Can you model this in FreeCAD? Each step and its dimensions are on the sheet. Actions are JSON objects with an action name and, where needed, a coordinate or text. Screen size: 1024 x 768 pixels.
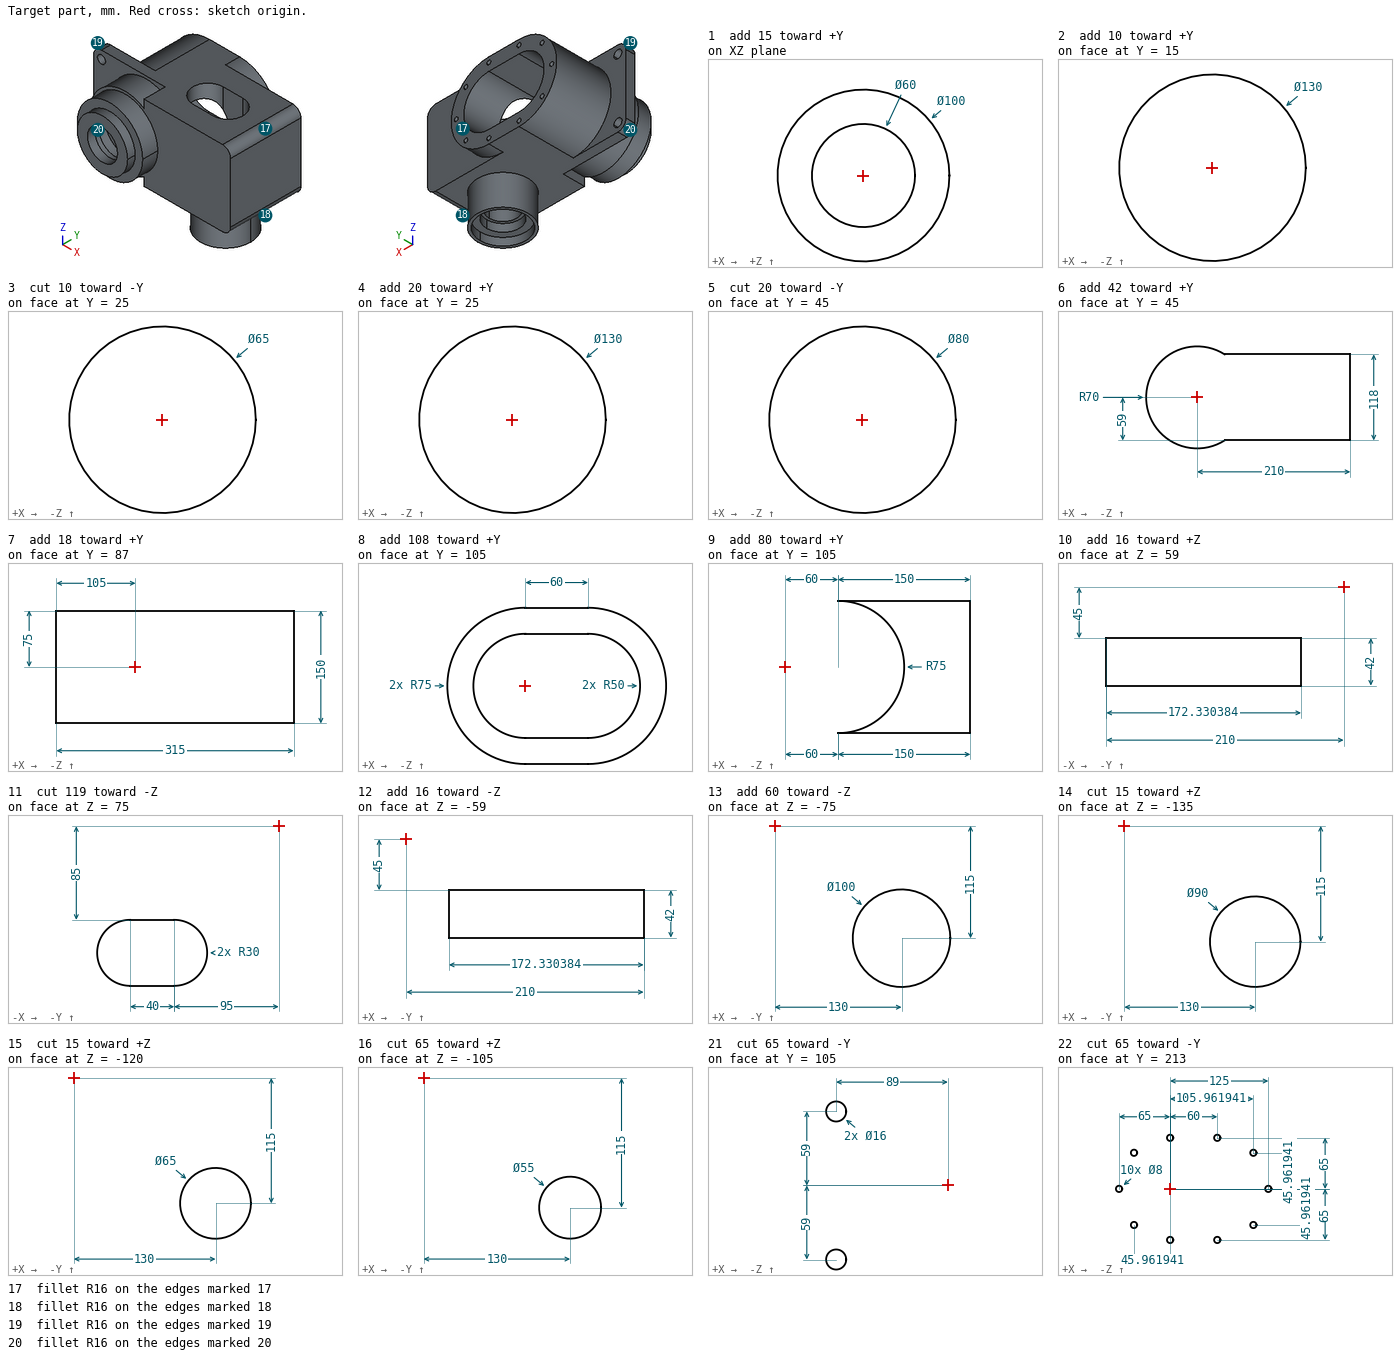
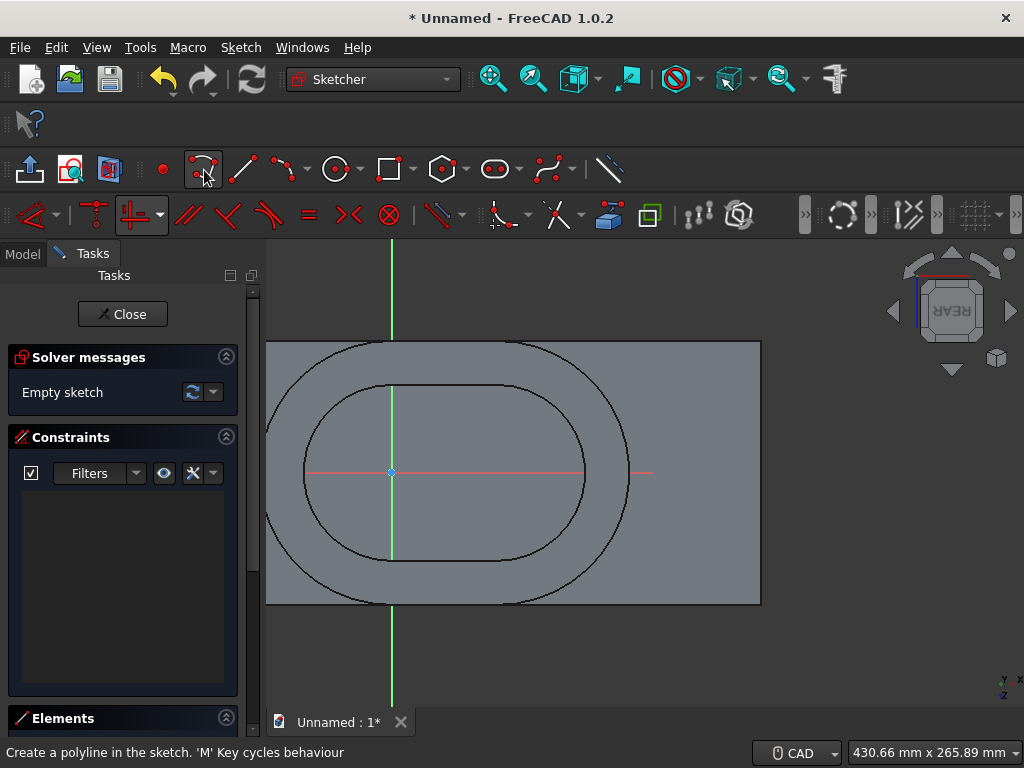
{"action": "left_click", "coordinate": [497, 605]}
{"action": "left_click", "coordinate": [761, 605]}
{"action": "left_click", "coordinate": [761, 341]}
{"action": "left_click", "coordinate": [497, 341]}
{"action": "right_click", "coordinate": [497, 341]}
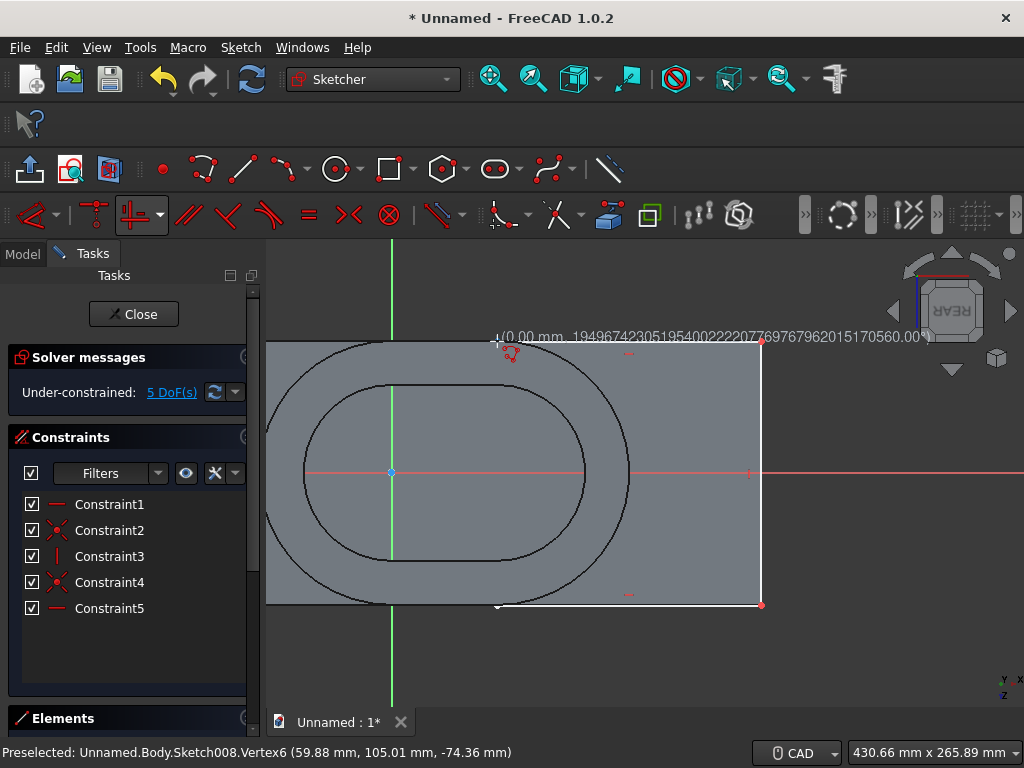
{"action": "left_click", "coordinate": [284, 170]}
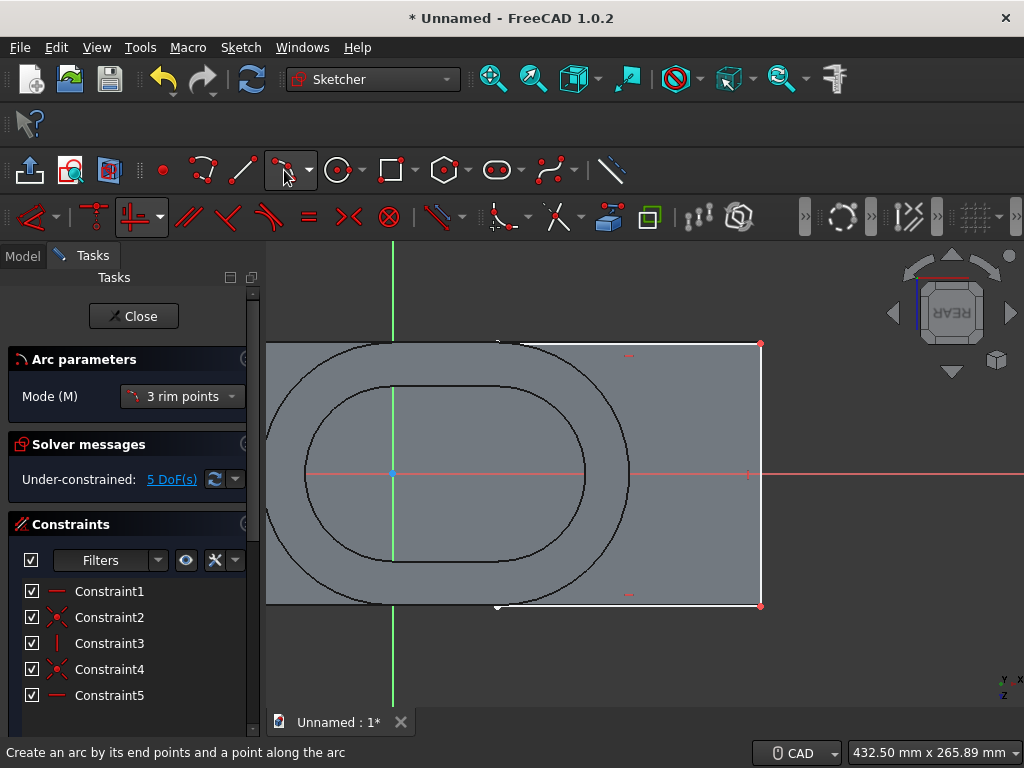
{"action": "left_click", "coordinate": [498, 344]}
{"action": "left_click", "coordinate": [498, 606]}
{"action": "left_click", "coordinate": [623, 515]}
{"action": "key", "text": "Escape"}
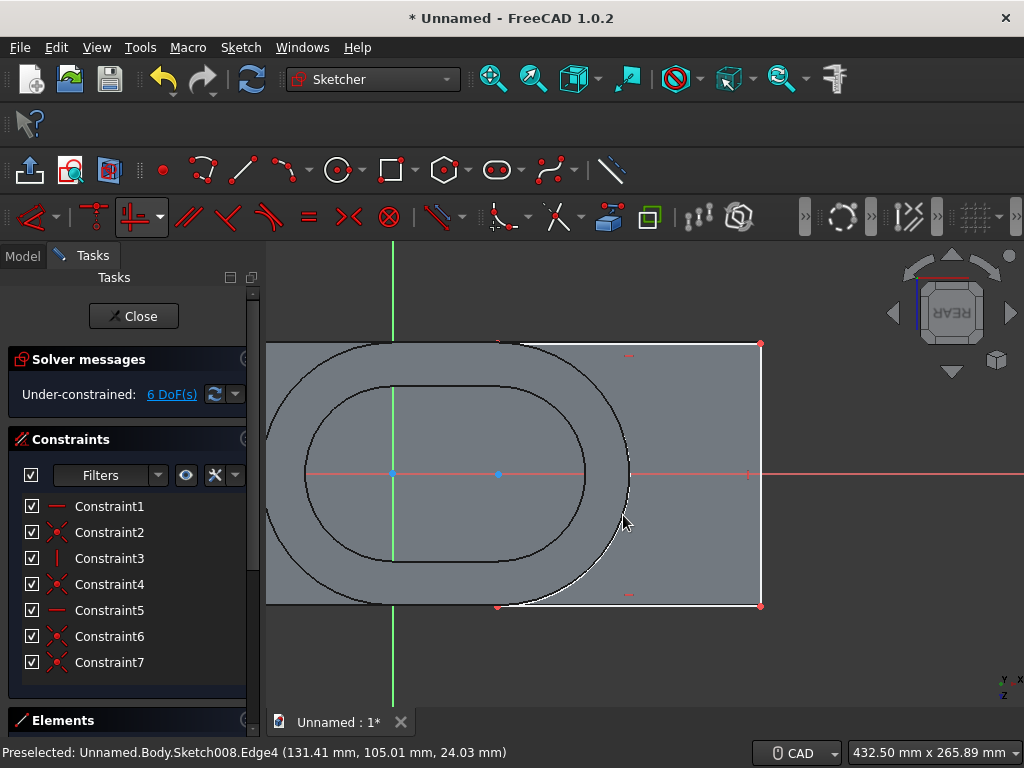
{"action": "left_click", "coordinate": [498, 475]}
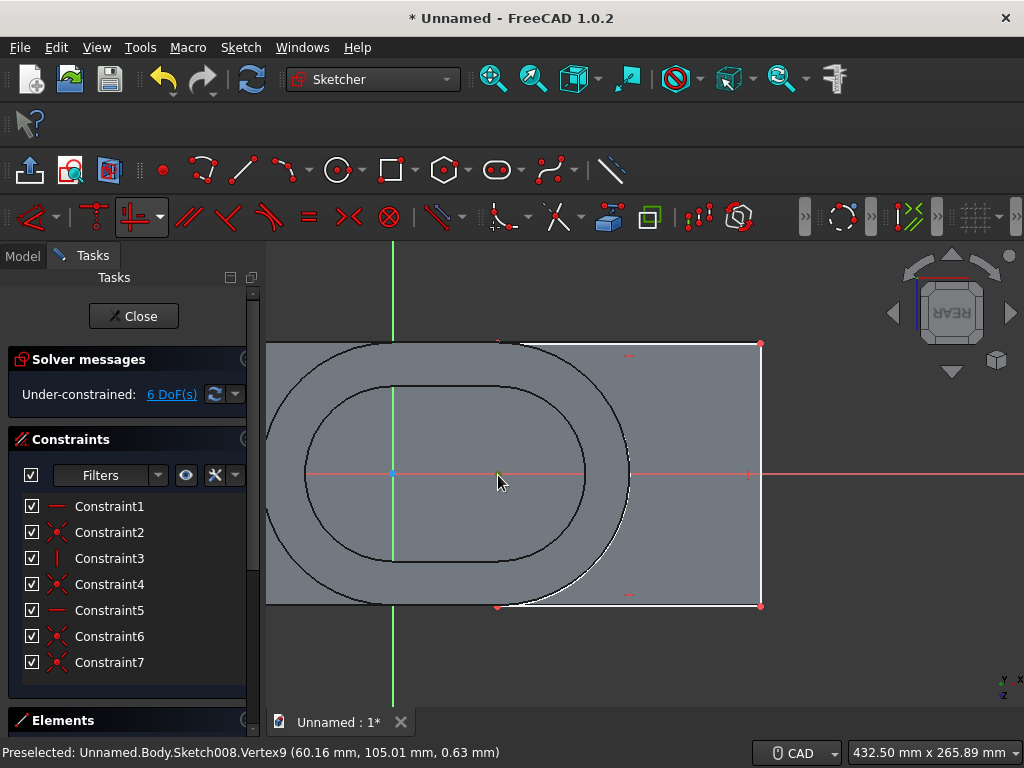
{"action": "left_click", "coordinate": [334, 474]}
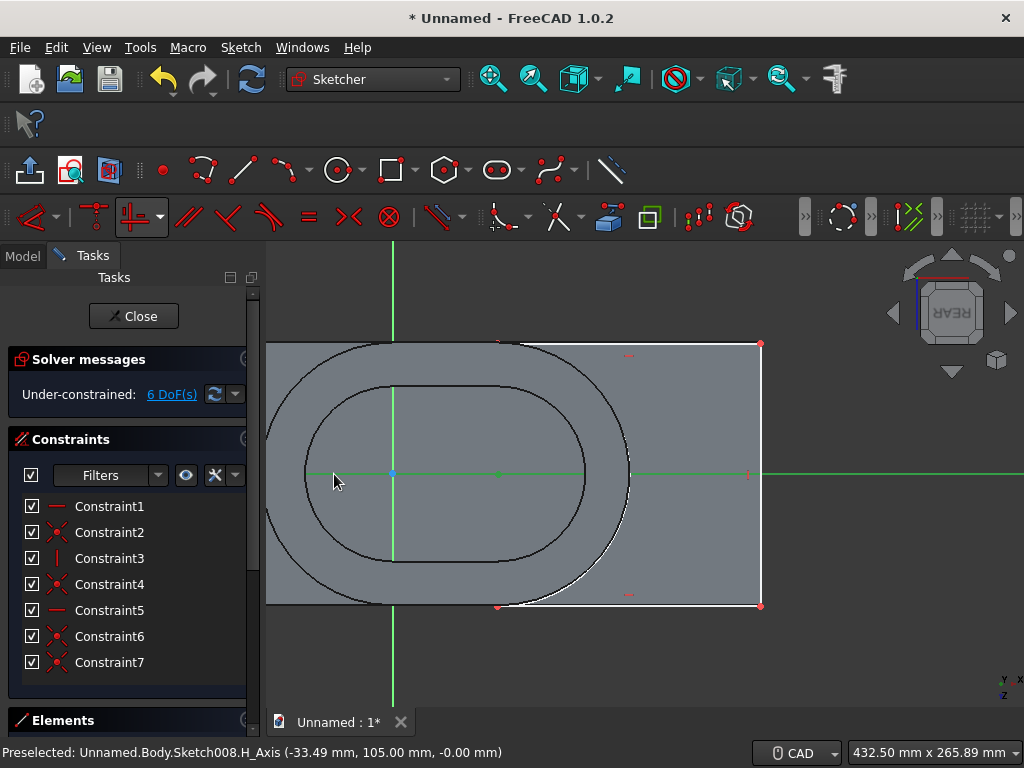
{"action": "left_click", "coordinate": [94, 218]}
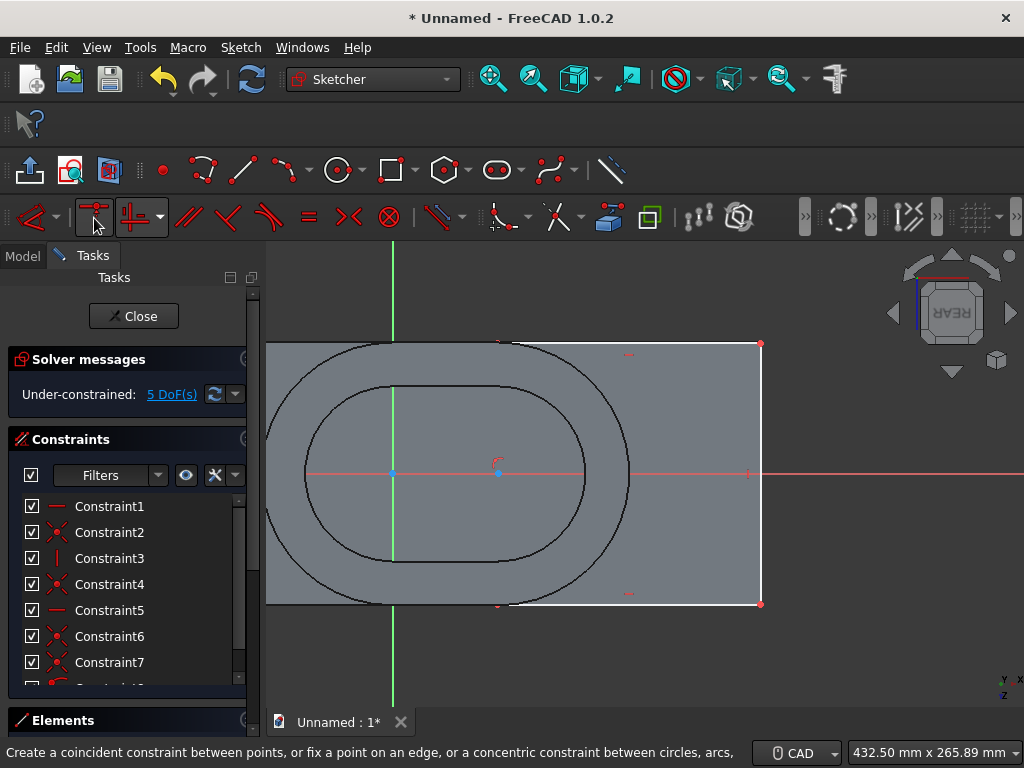
{"action": "left_click", "coordinate": [32, 218]}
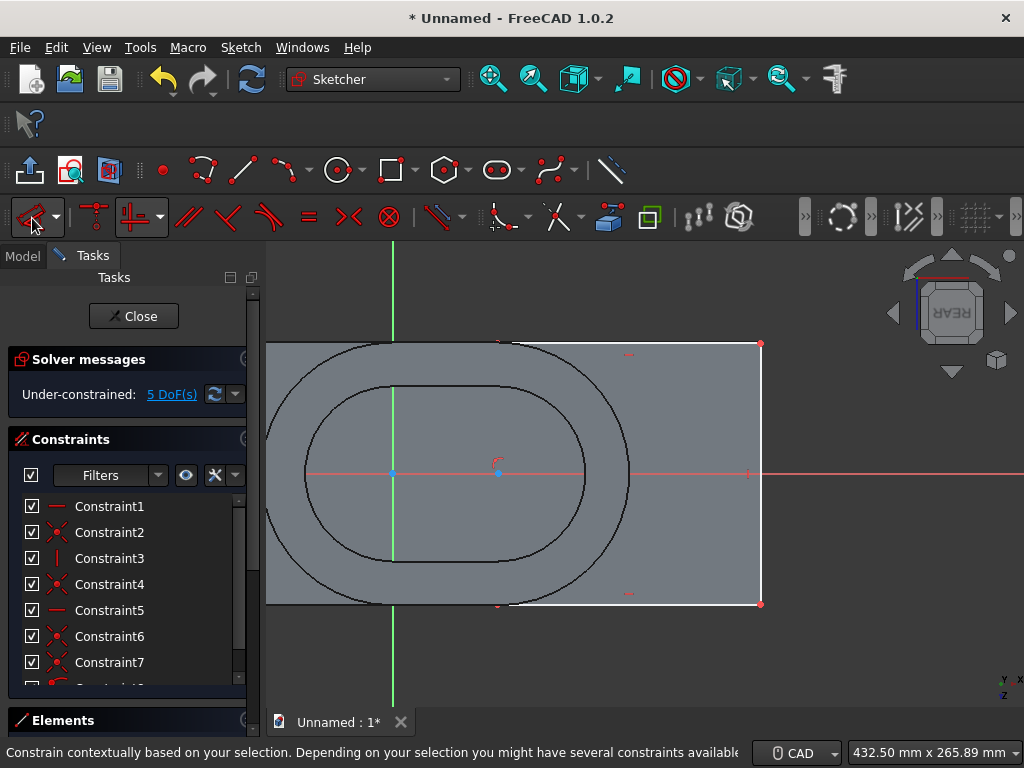
{"action": "left_click", "coordinate": [604, 551]}
{"action": "left_click", "coordinate": [630, 570]}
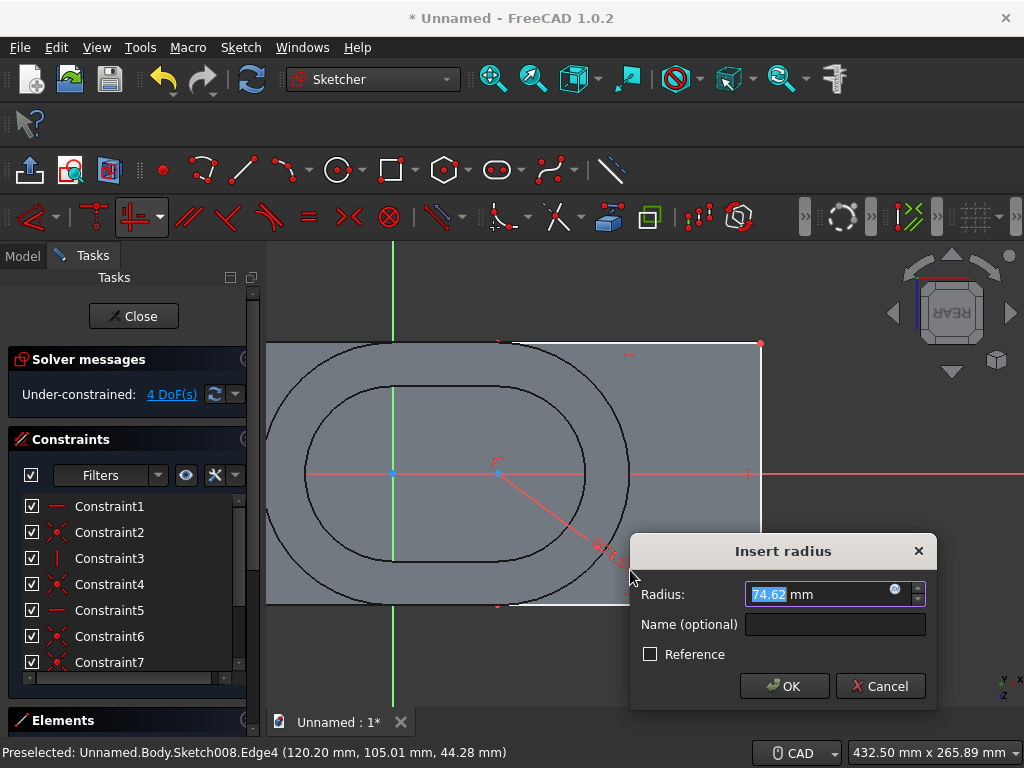
{"action": "type", "text": "75"}
{"action": "key", "text": "Return"}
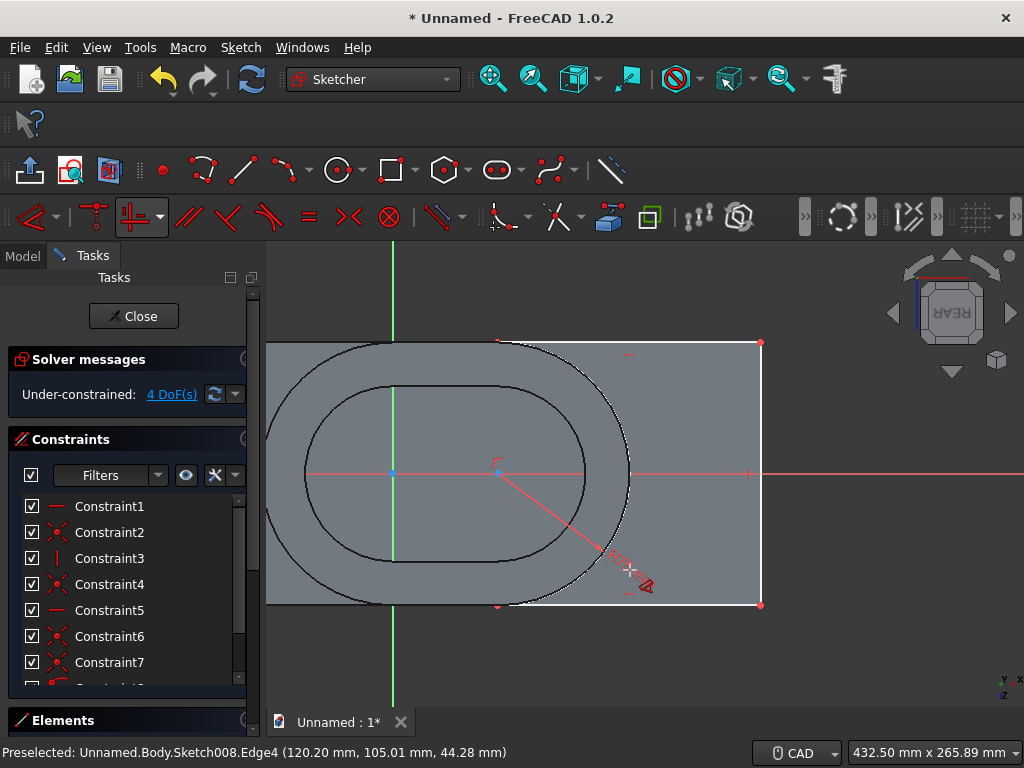
{"action": "left_click", "coordinate": [576, 605]}
{"action": "left_click", "coordinate": [629, 639]}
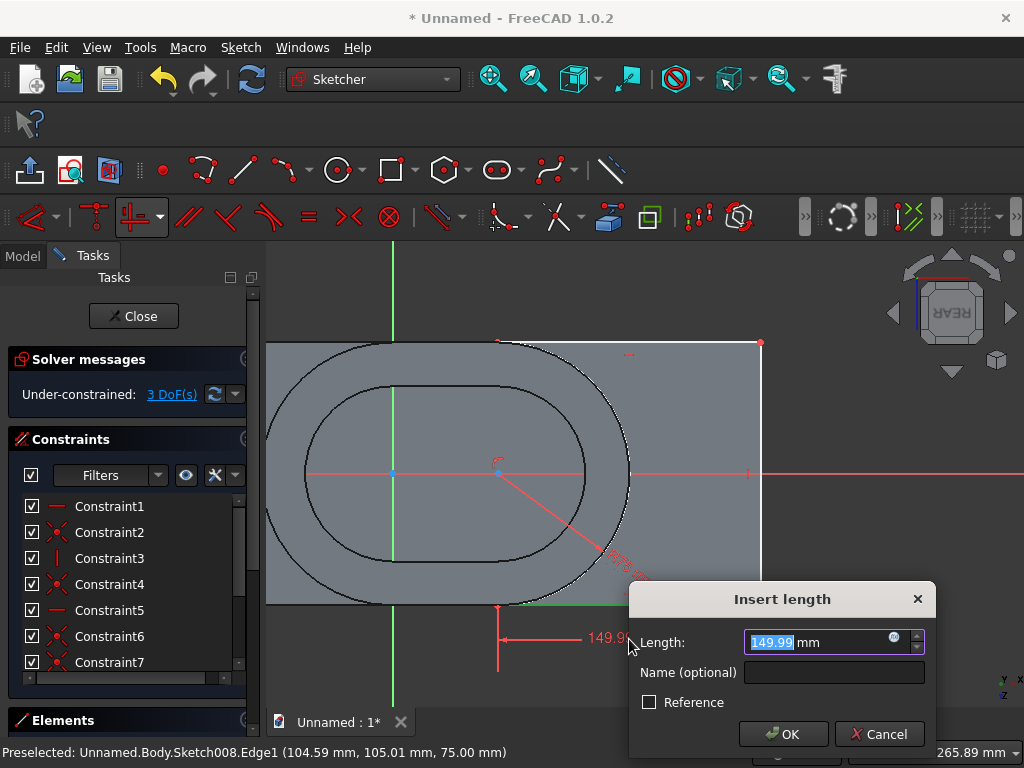
{"action": "type", "text": "150"}
{"action": "key", "text": "Return"}